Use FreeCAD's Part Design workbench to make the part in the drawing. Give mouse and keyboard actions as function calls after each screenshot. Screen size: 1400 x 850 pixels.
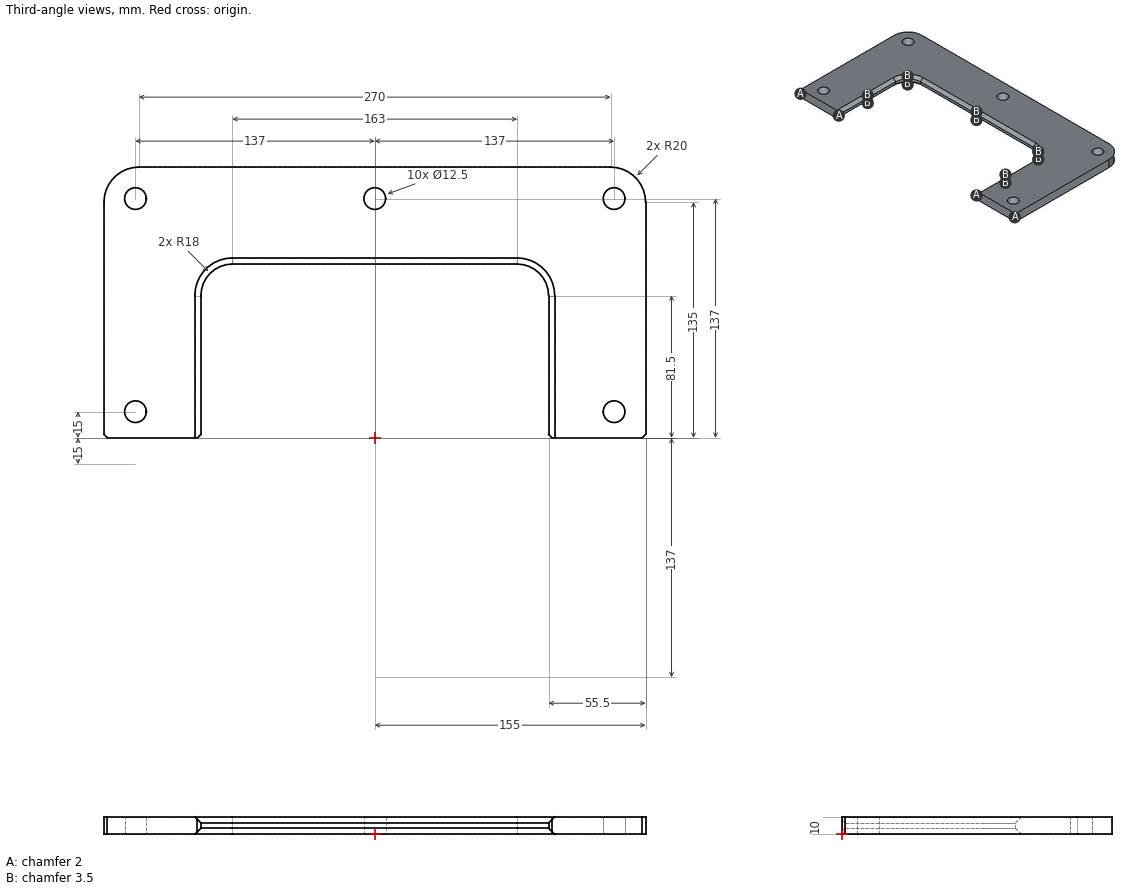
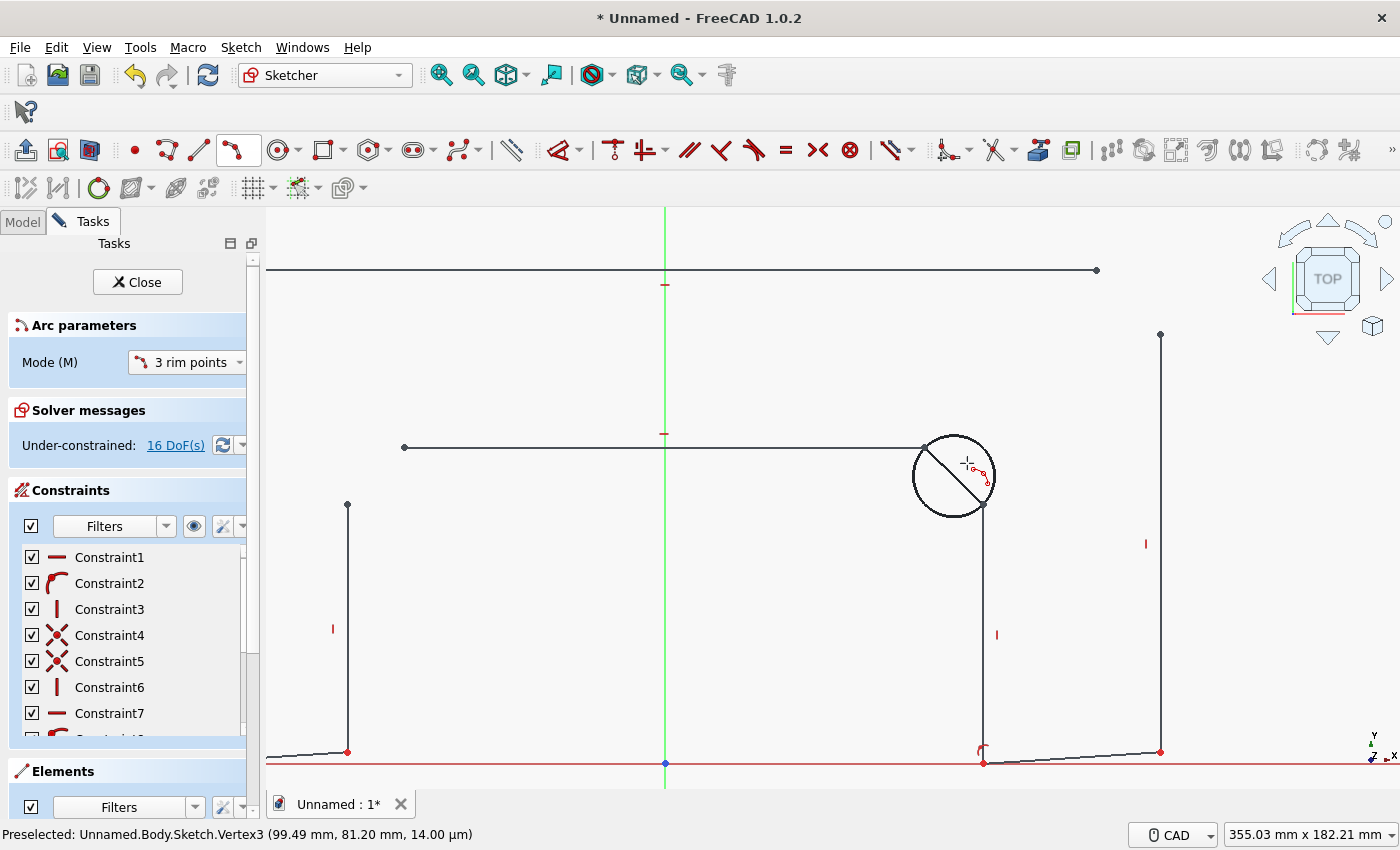
click(966, 463)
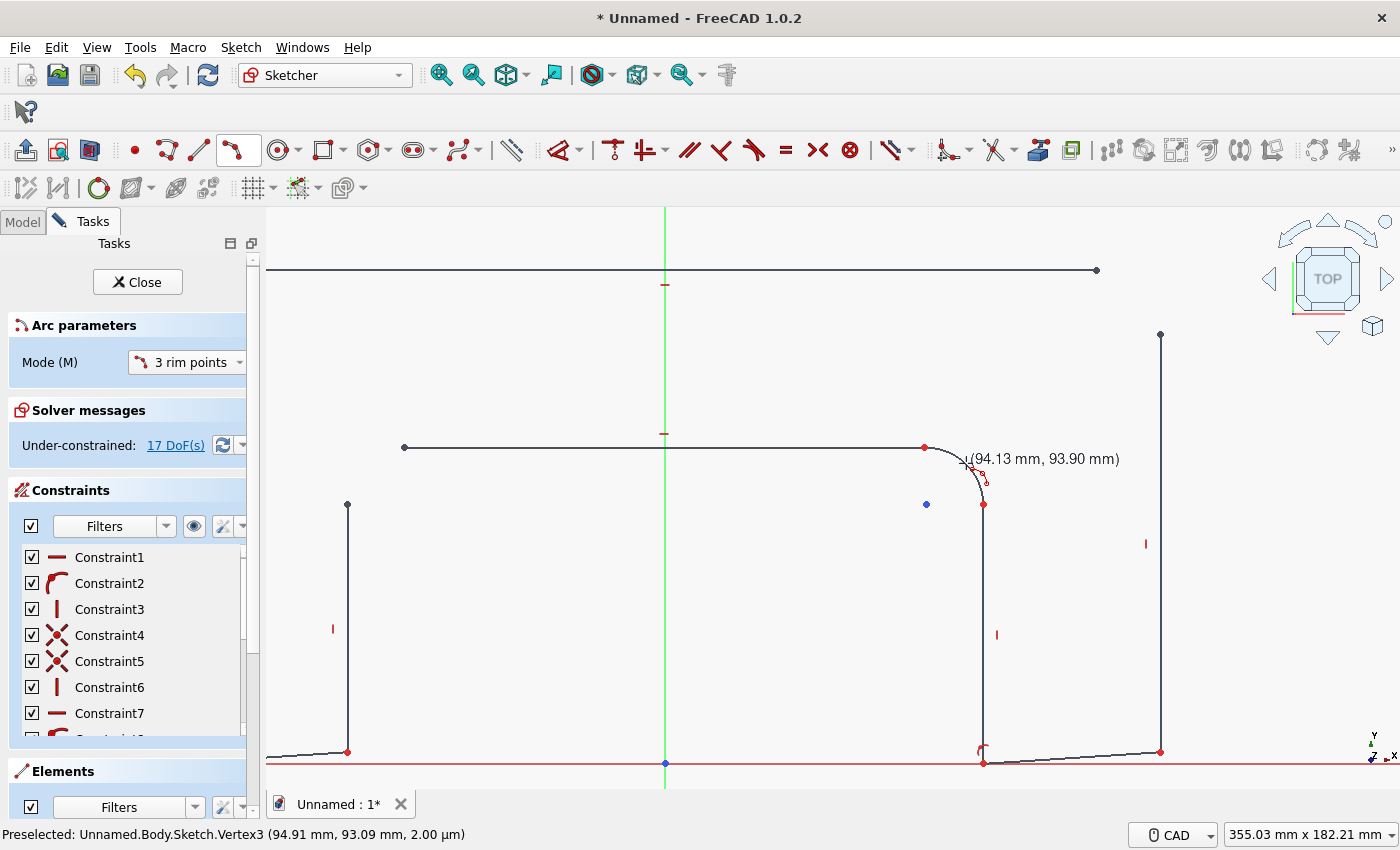
click(1161, 334)
click(1096, 270)
click(1142, 288)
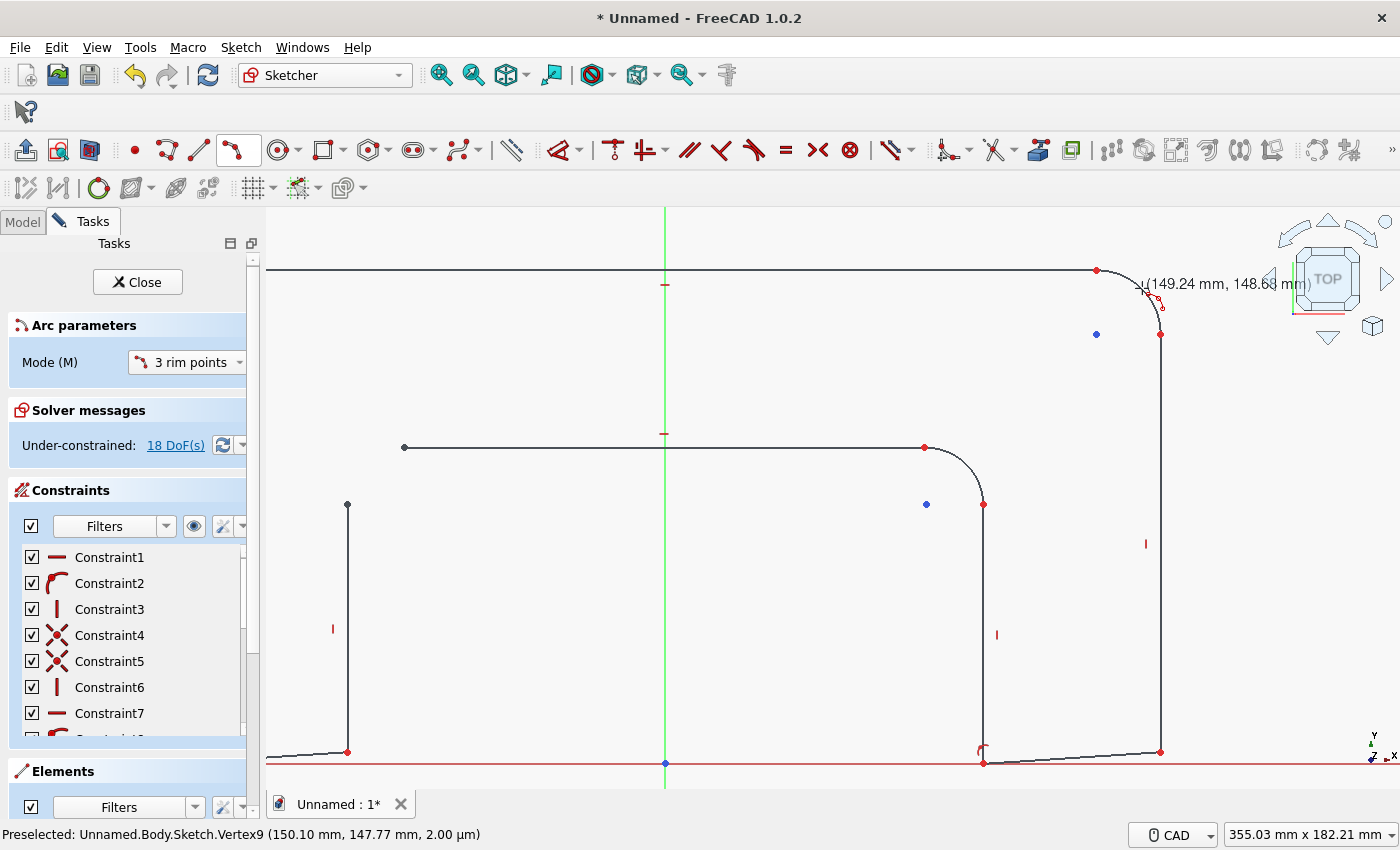
scroll(966, 461, down, 2)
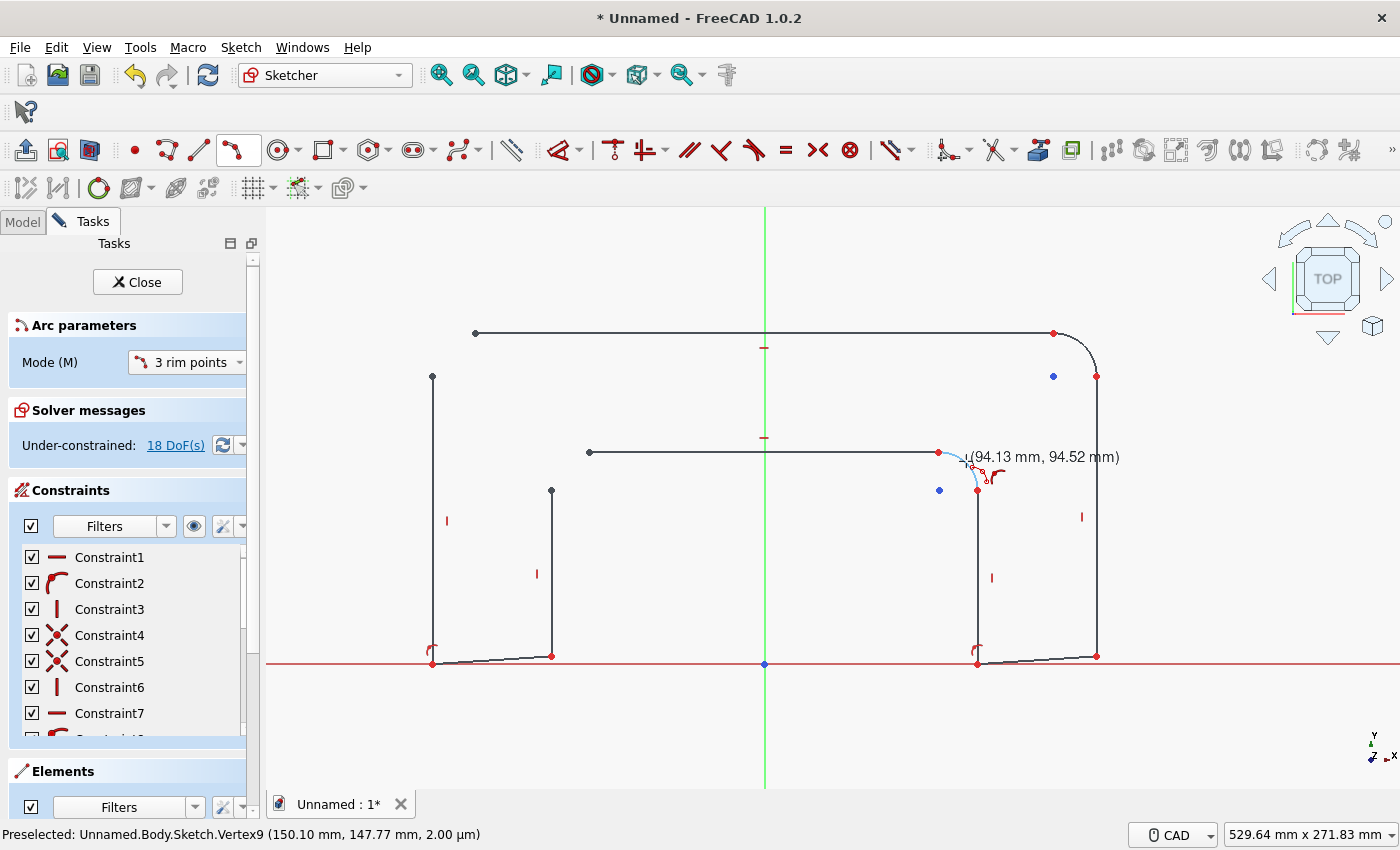
click(476, 333)
click(433, 376)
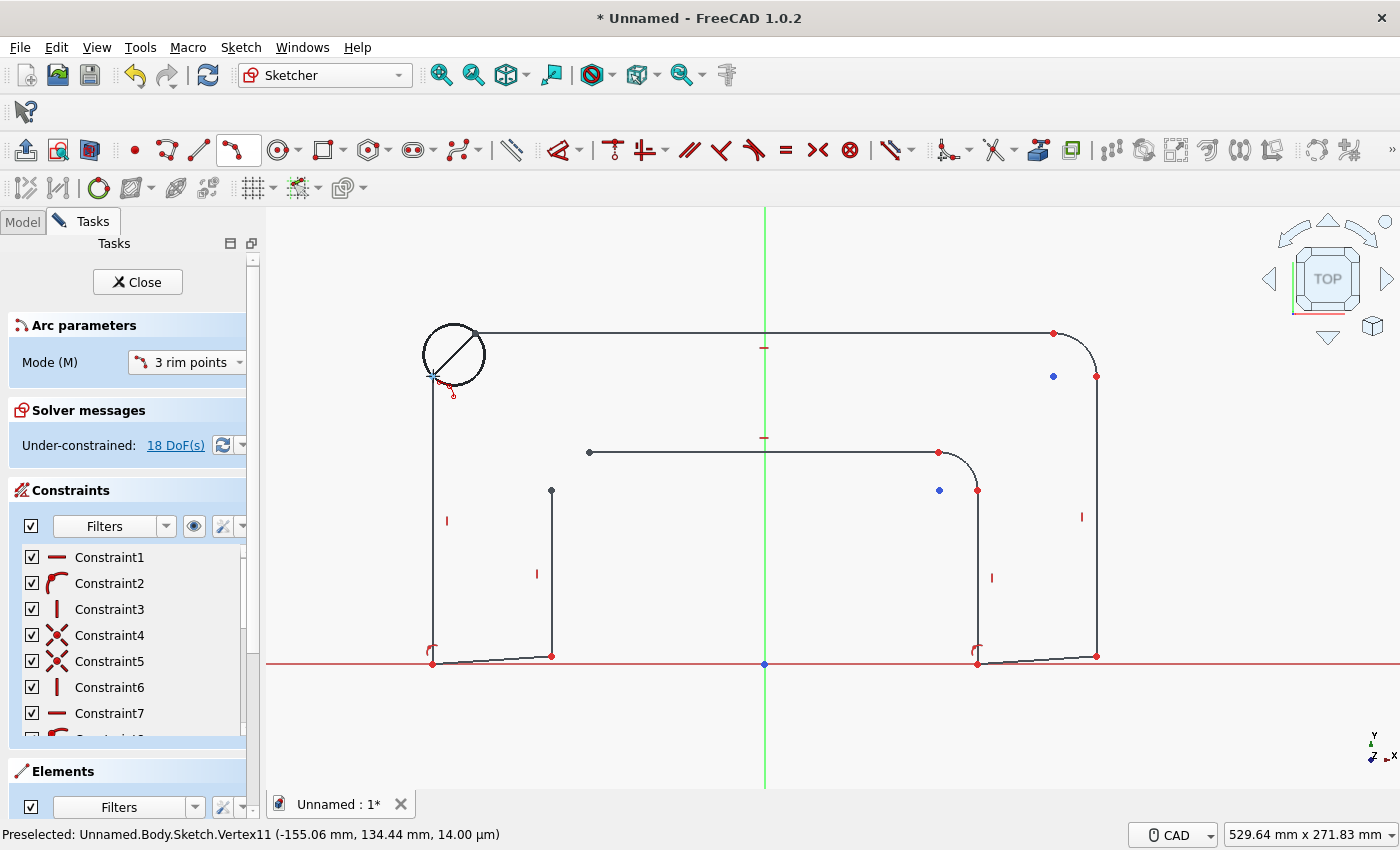
scroll(445, 345, up, 2)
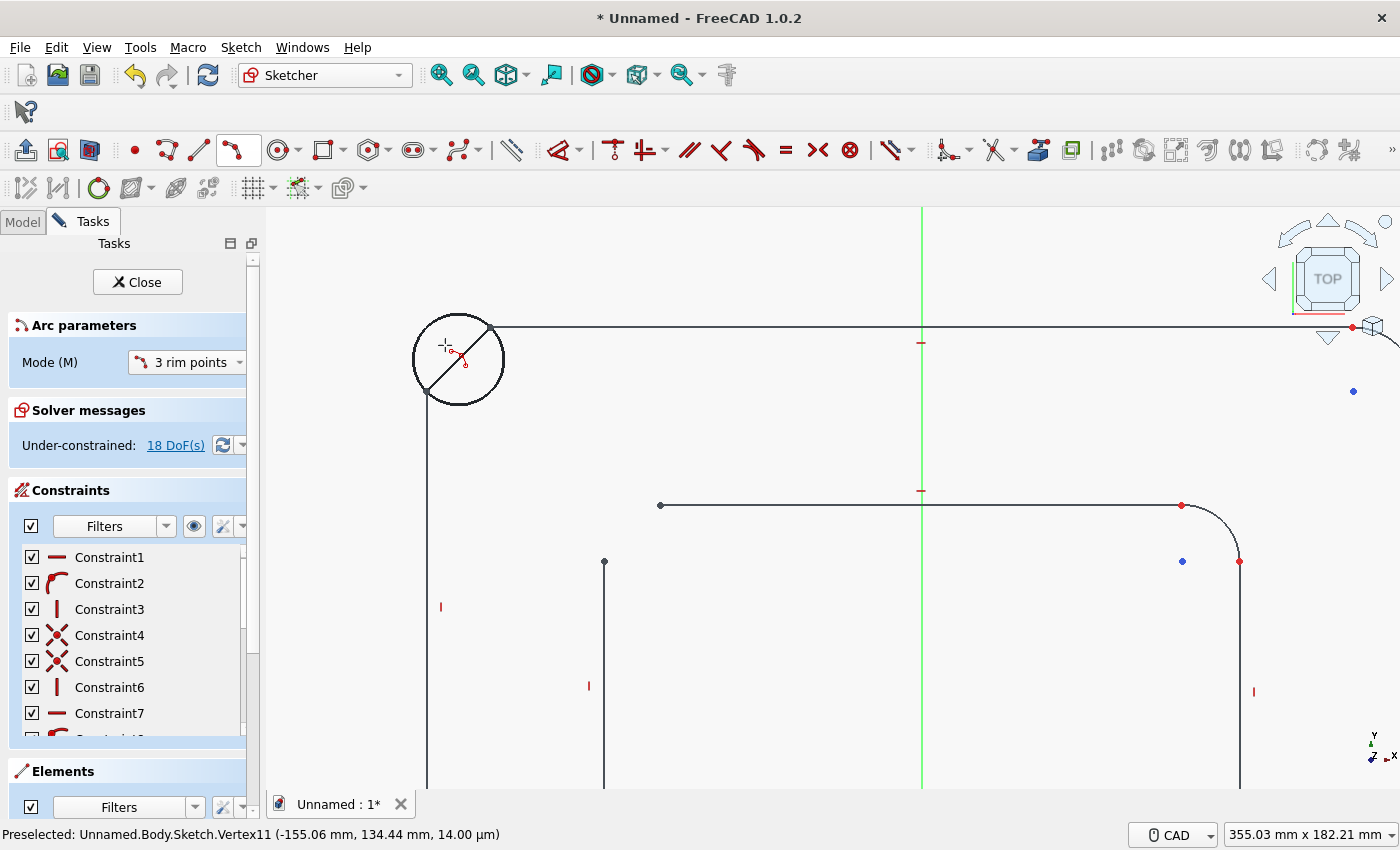
click(445, 345)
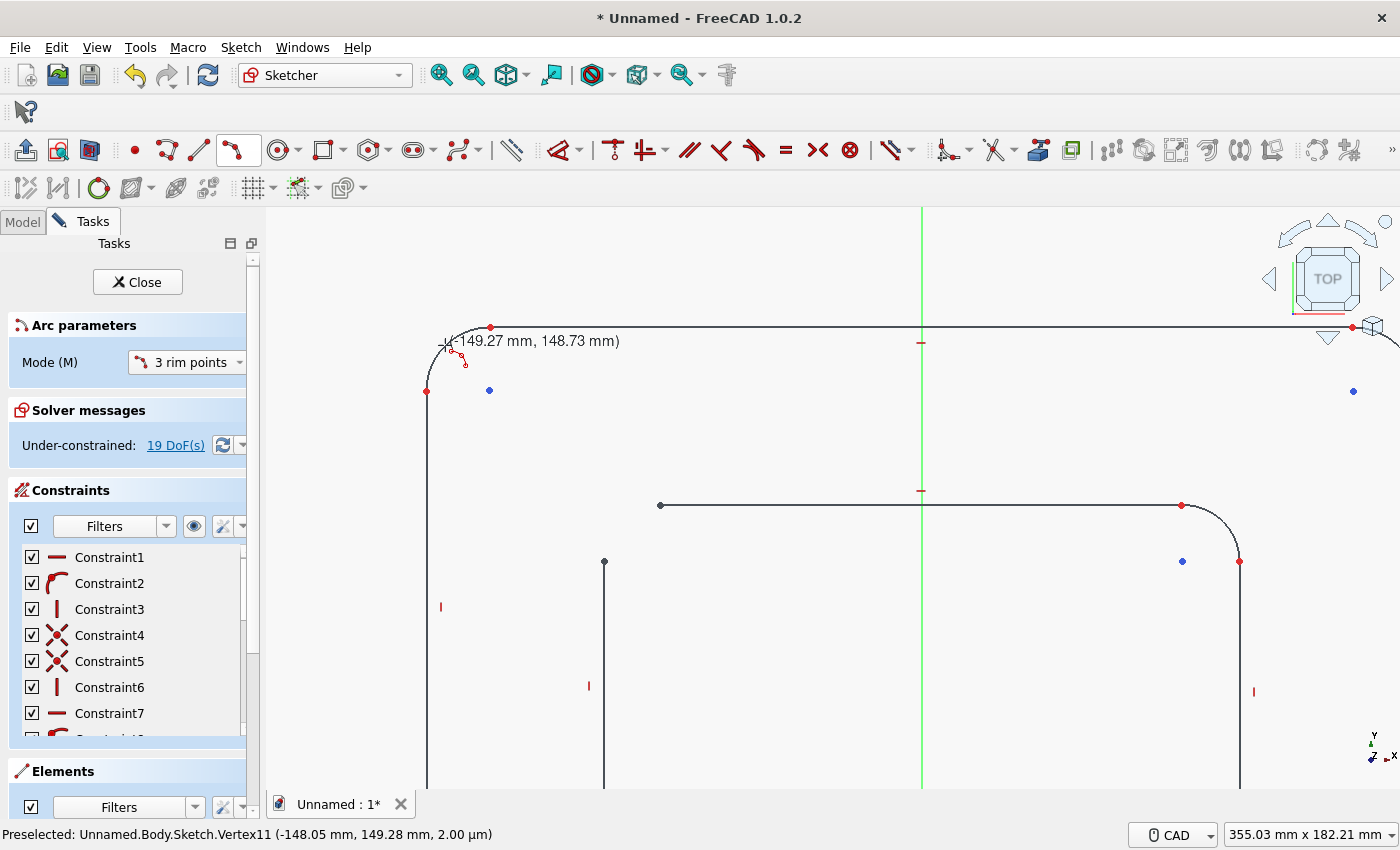
click(604, 562)
click(661, 505)
click(621, 520)
key(Escape)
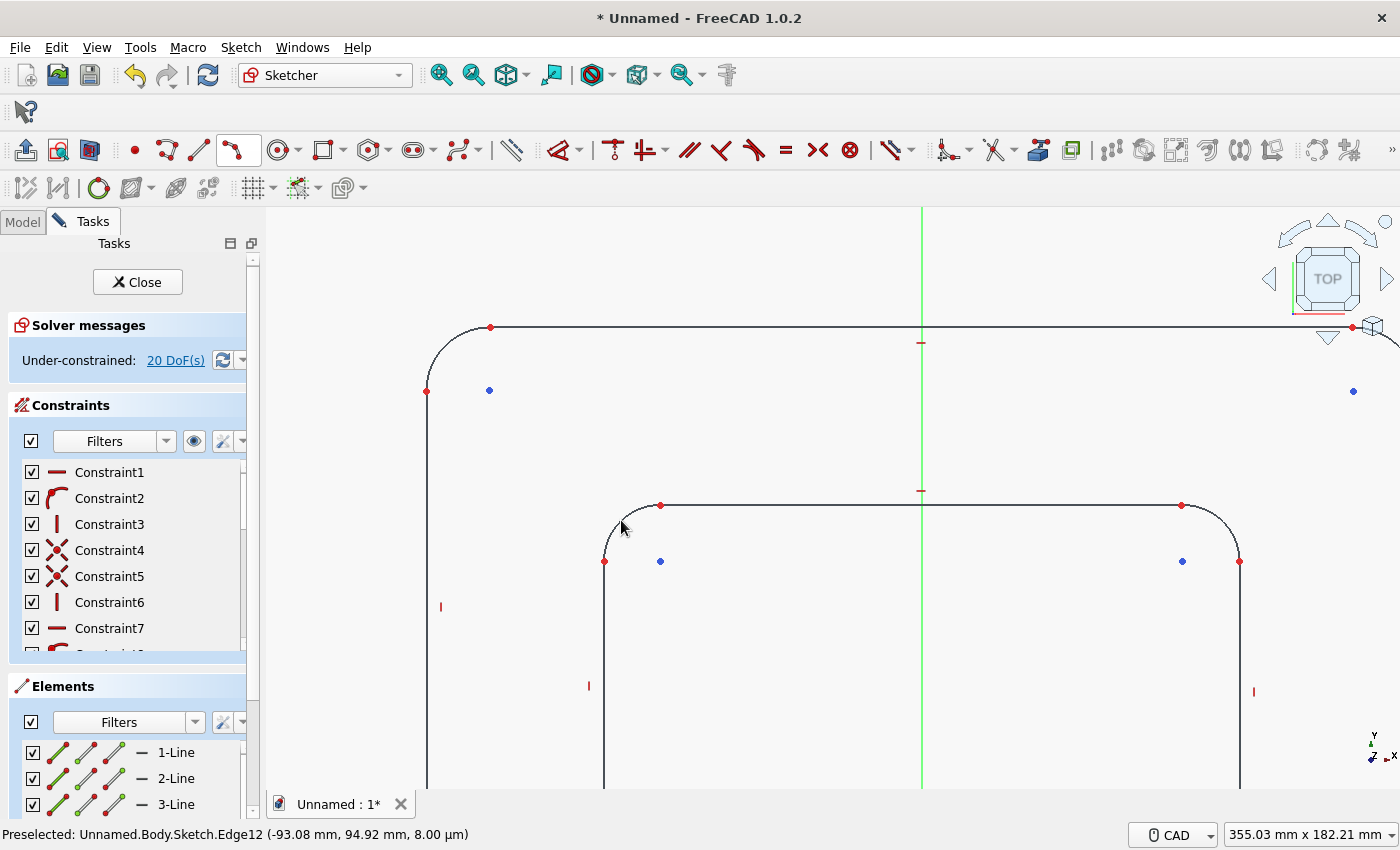
click(817, 505)